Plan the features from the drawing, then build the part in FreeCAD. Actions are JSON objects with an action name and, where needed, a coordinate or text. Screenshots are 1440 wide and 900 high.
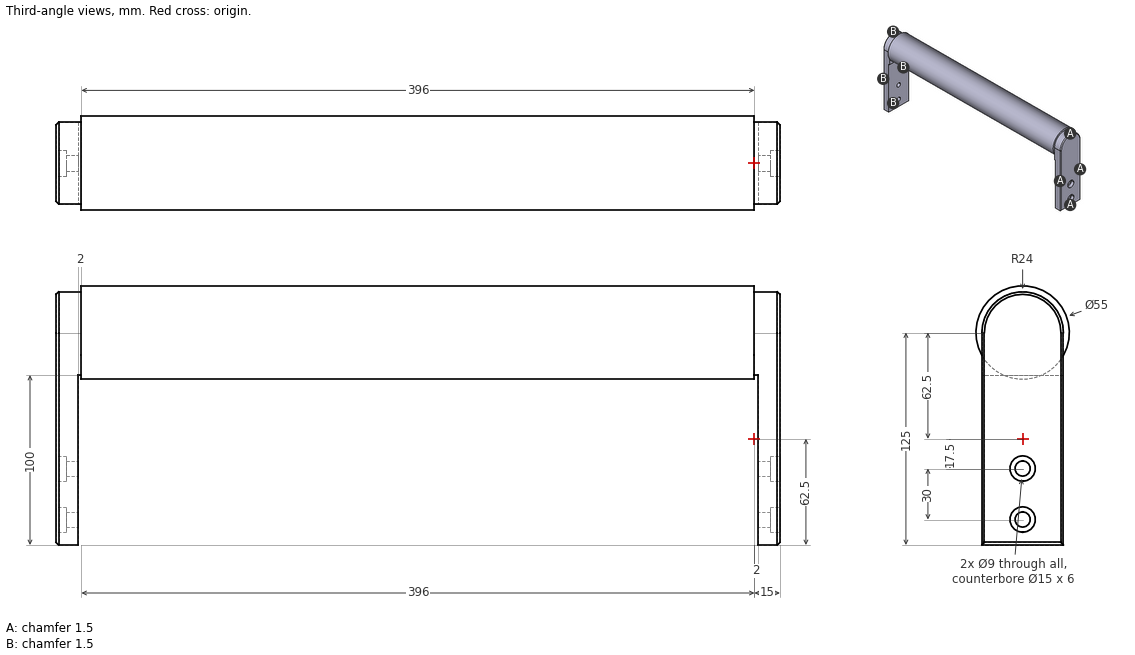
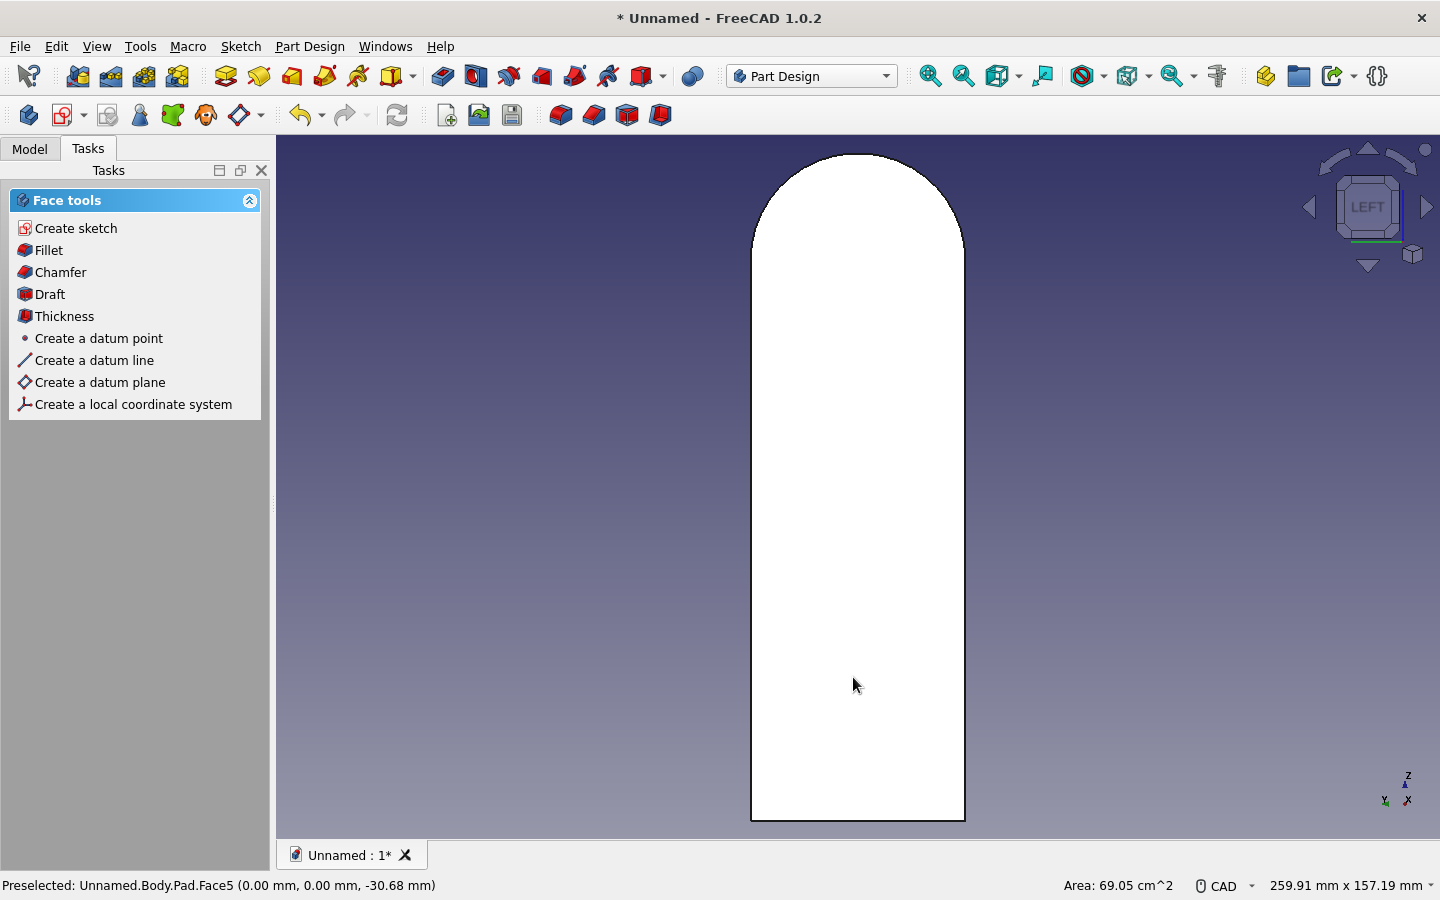
{"action": "left_click", "coordinate": [62, 116]}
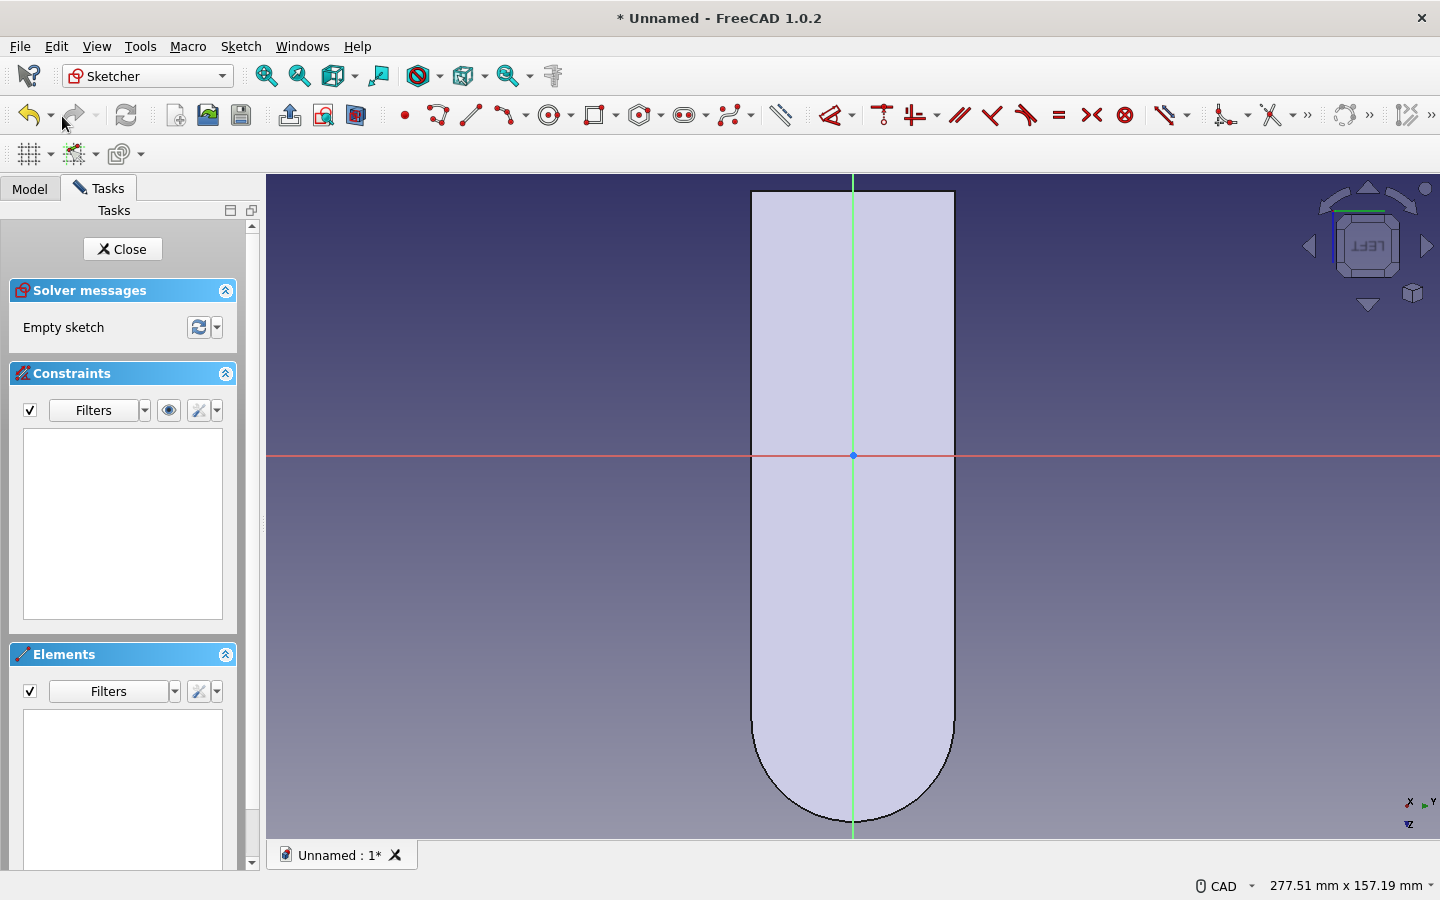
{"action": "scroll", "coordinate": [475, 202], "scroll_direction": "down", "scroll_amount": 1}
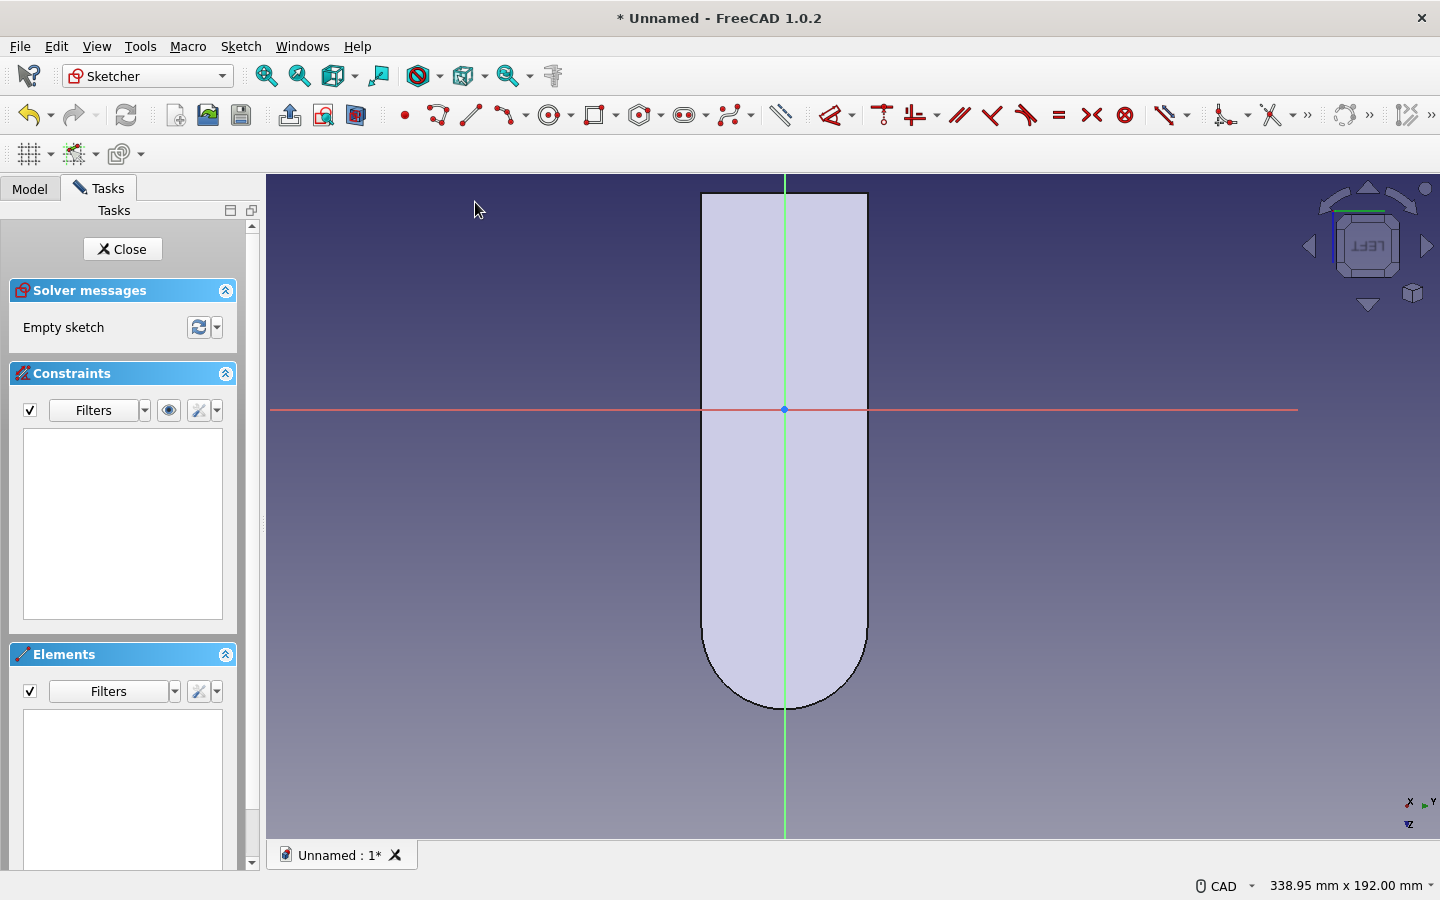
{"action": "scroll", "coordinate": [785, 686], "scroll_direction": "up", "scroll_amount": 2}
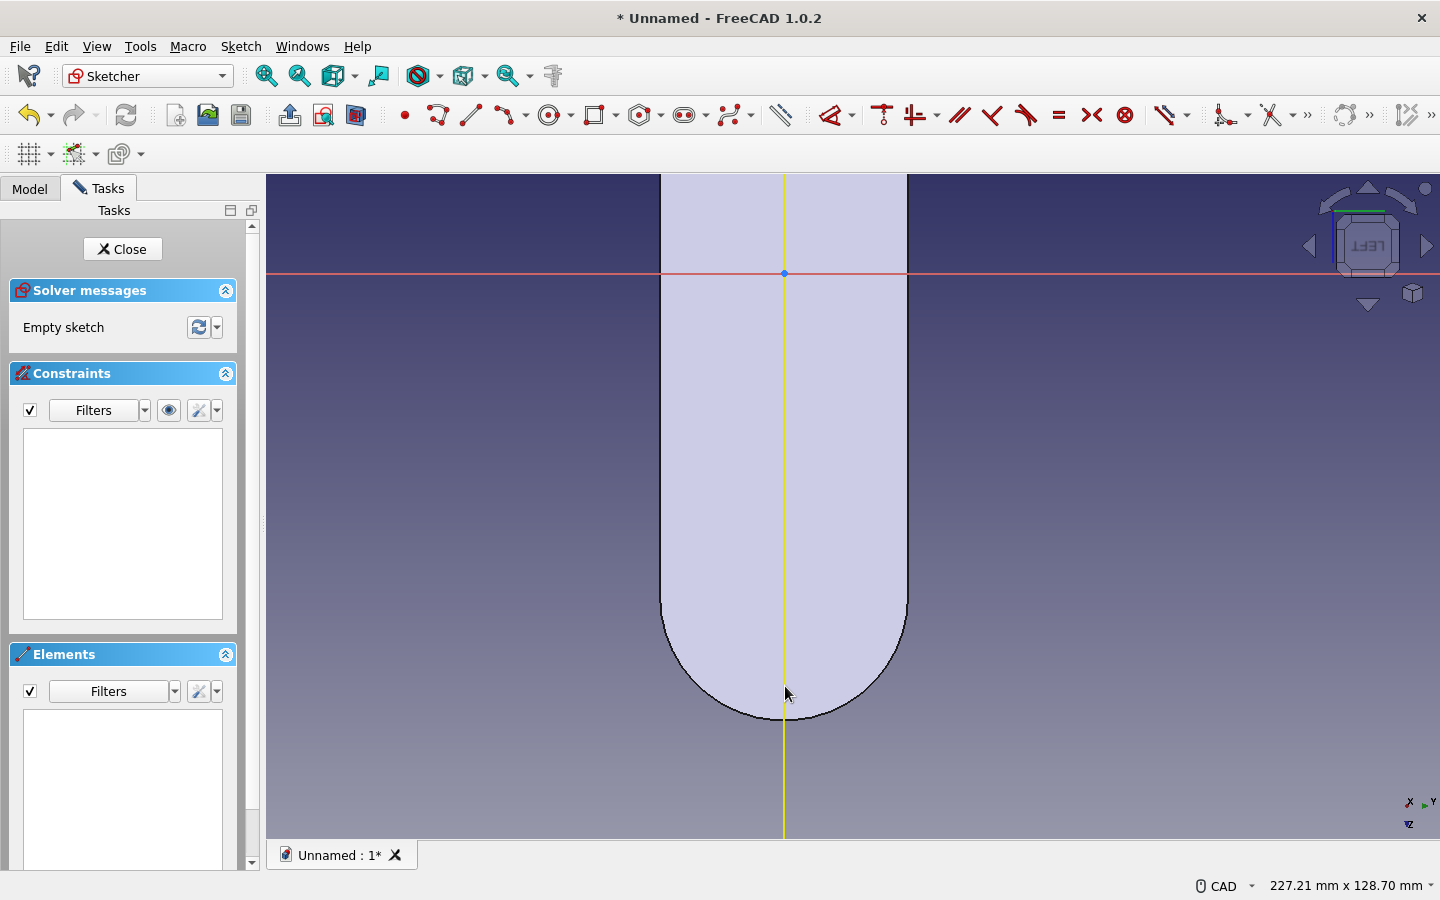
{"action": "left_click", "coordinate": [548, 116]}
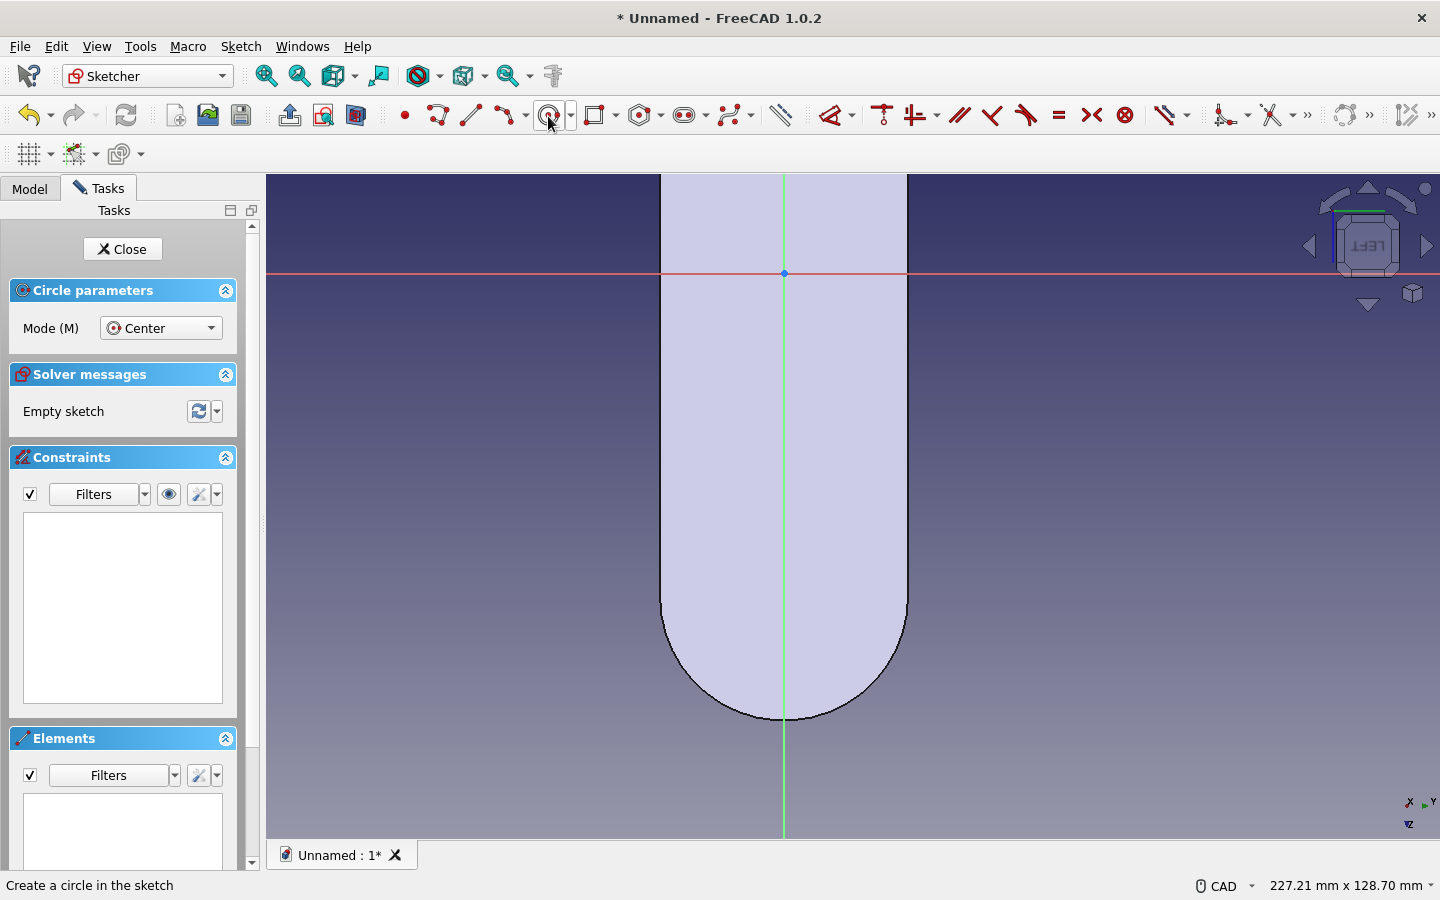
{"action": "left_click", "coordinate": [784, 597]}
{"action": "mouse_move", "coordinate": [885, 496]}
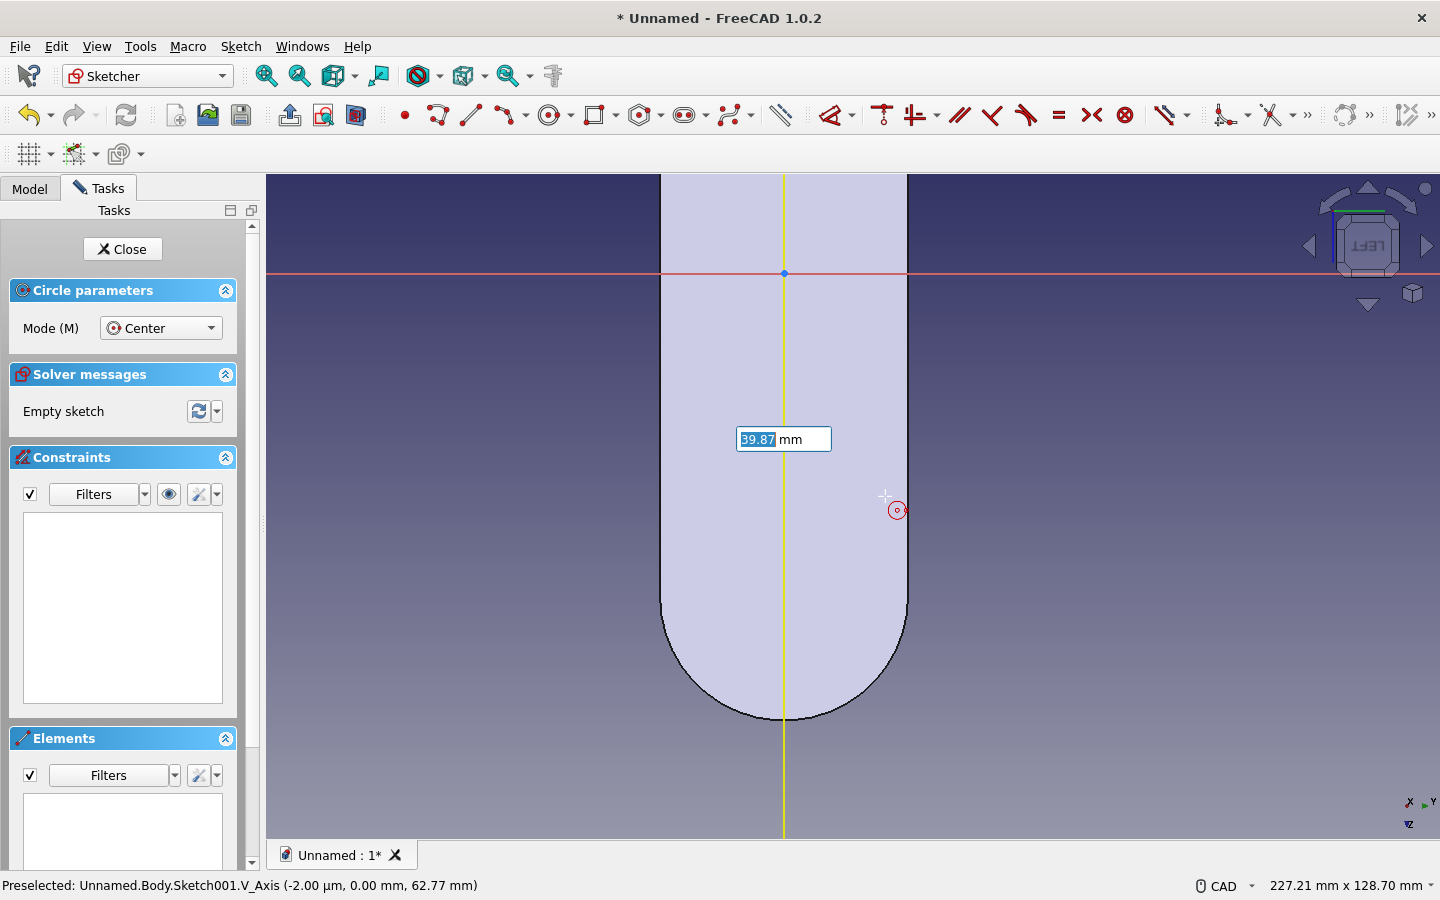
{"action": "type", "text": "55"}
{"action": "key", "text": "Return"}
{"action": "key", "text": "Escape"}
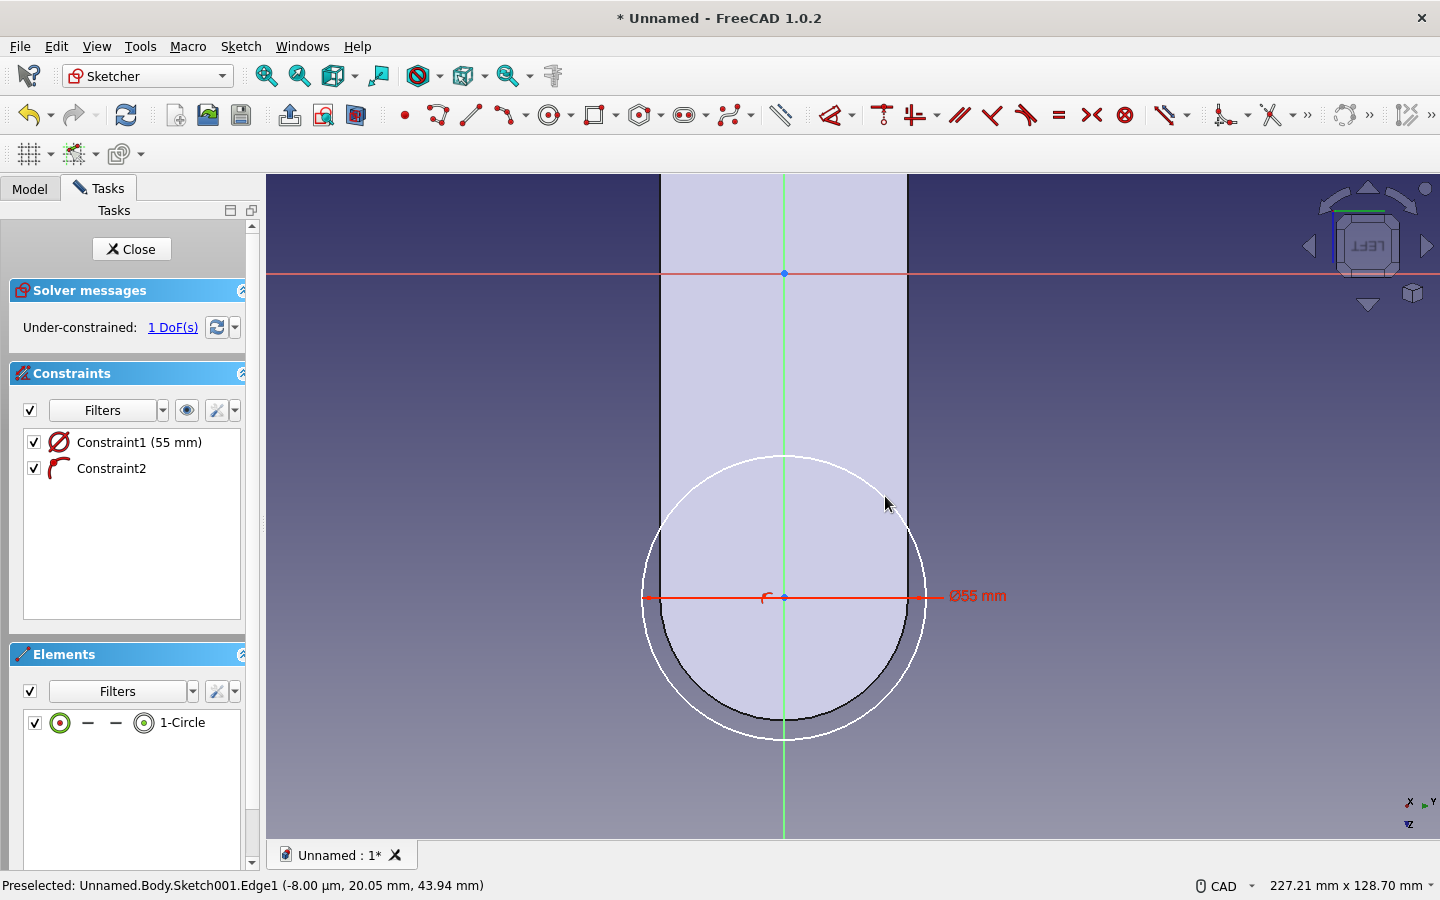
{"action": "left_click", "coordinate": [830, 116]}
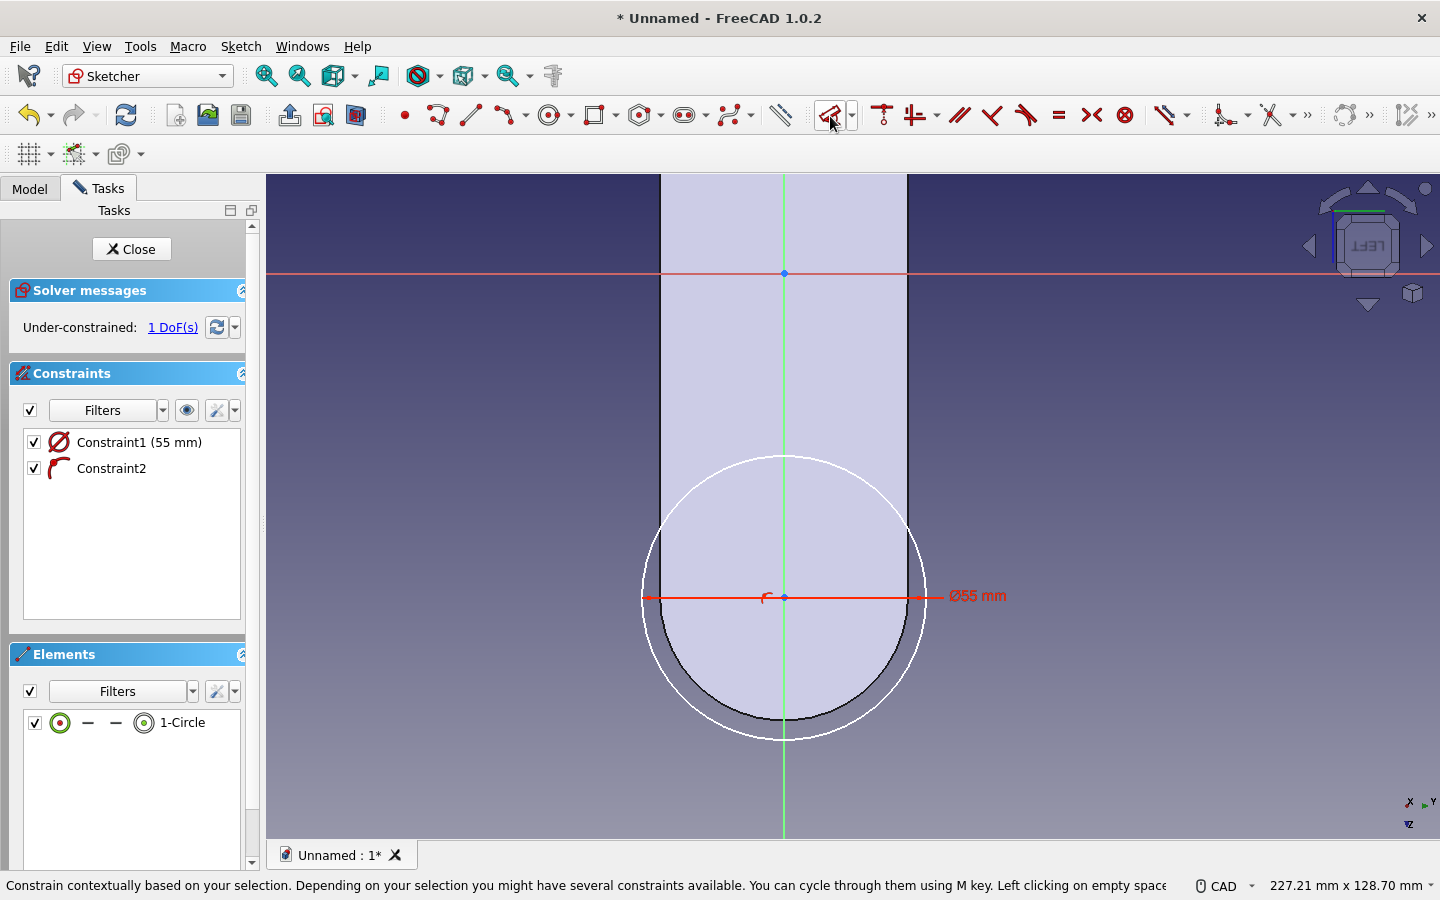
{"action": "left_click", "coordinate": [784, 598]}
{"action": "left_click", "coordinate": [818, 436]}